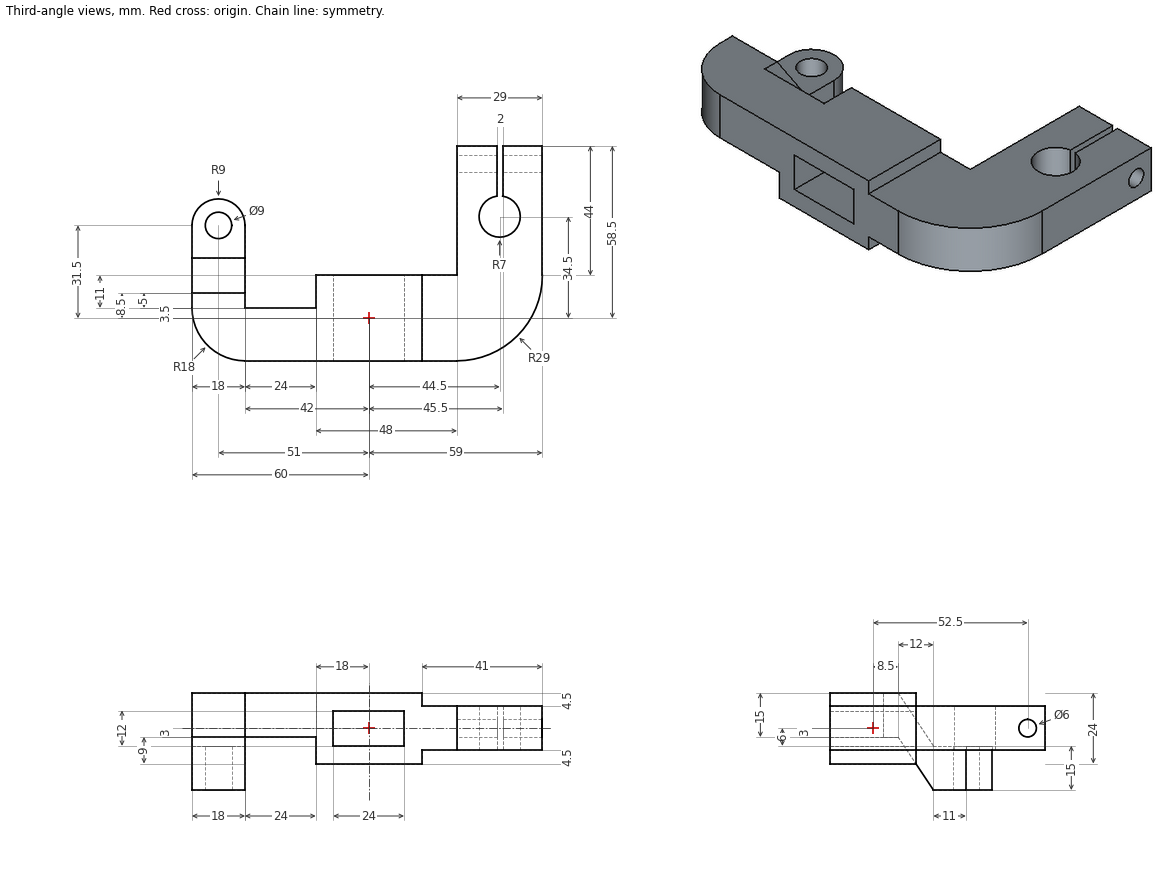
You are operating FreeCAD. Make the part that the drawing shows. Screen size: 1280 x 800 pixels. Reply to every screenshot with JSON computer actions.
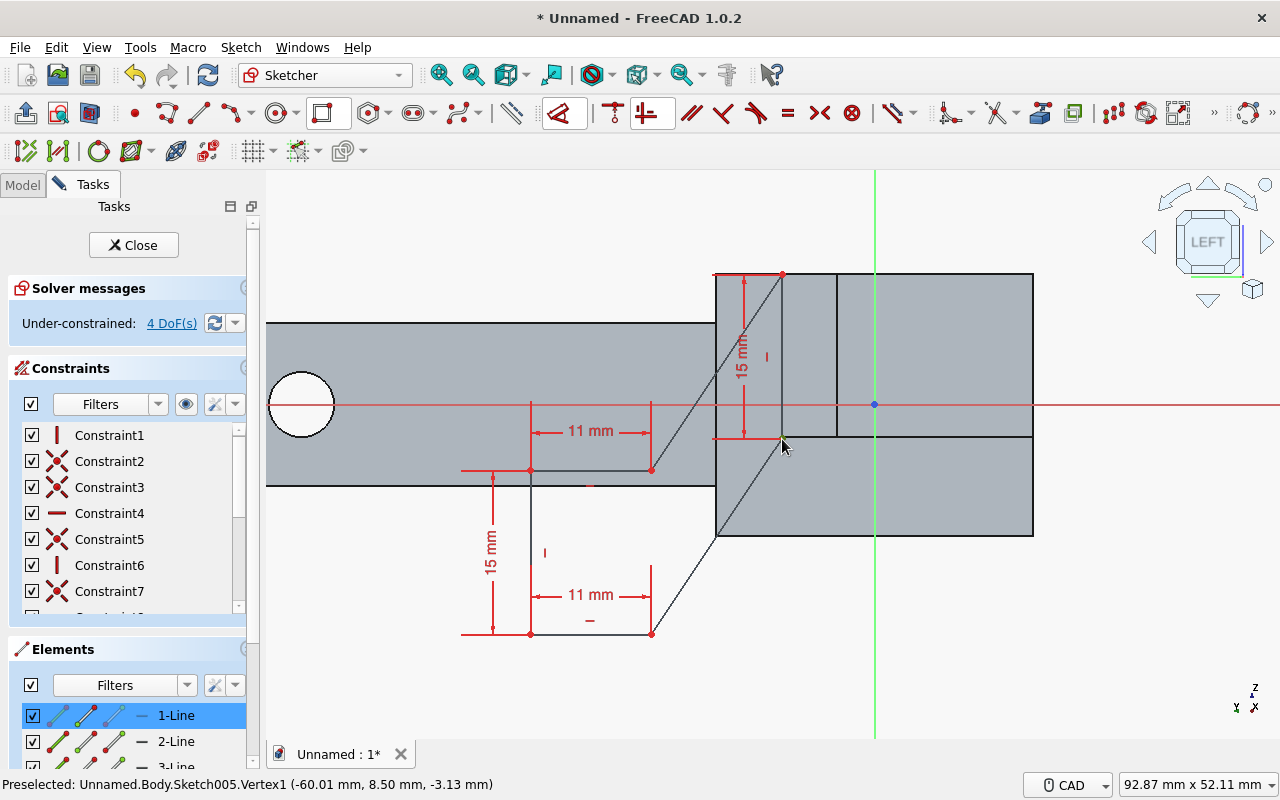
{"action": "key", "text": "i"}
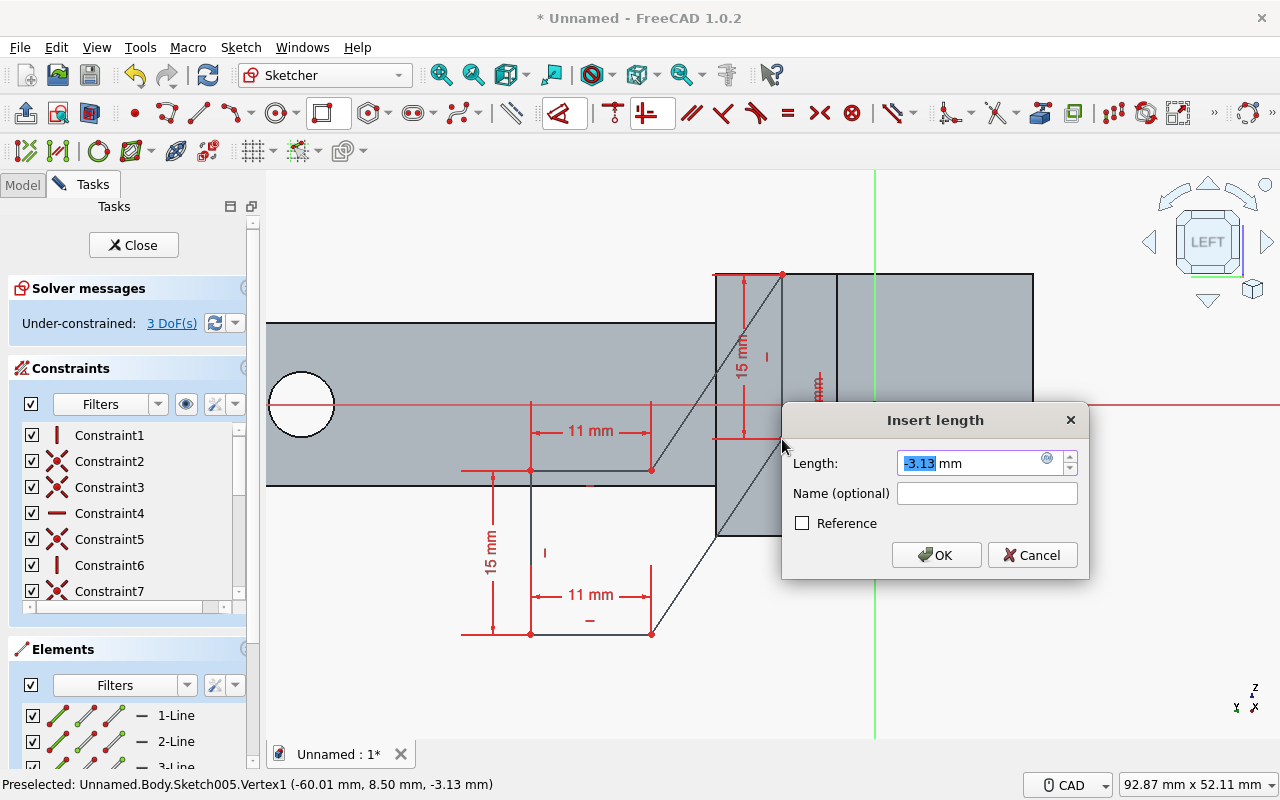
{"action": "type", "text": "-3"}
{"action": "key", "text": "Return"}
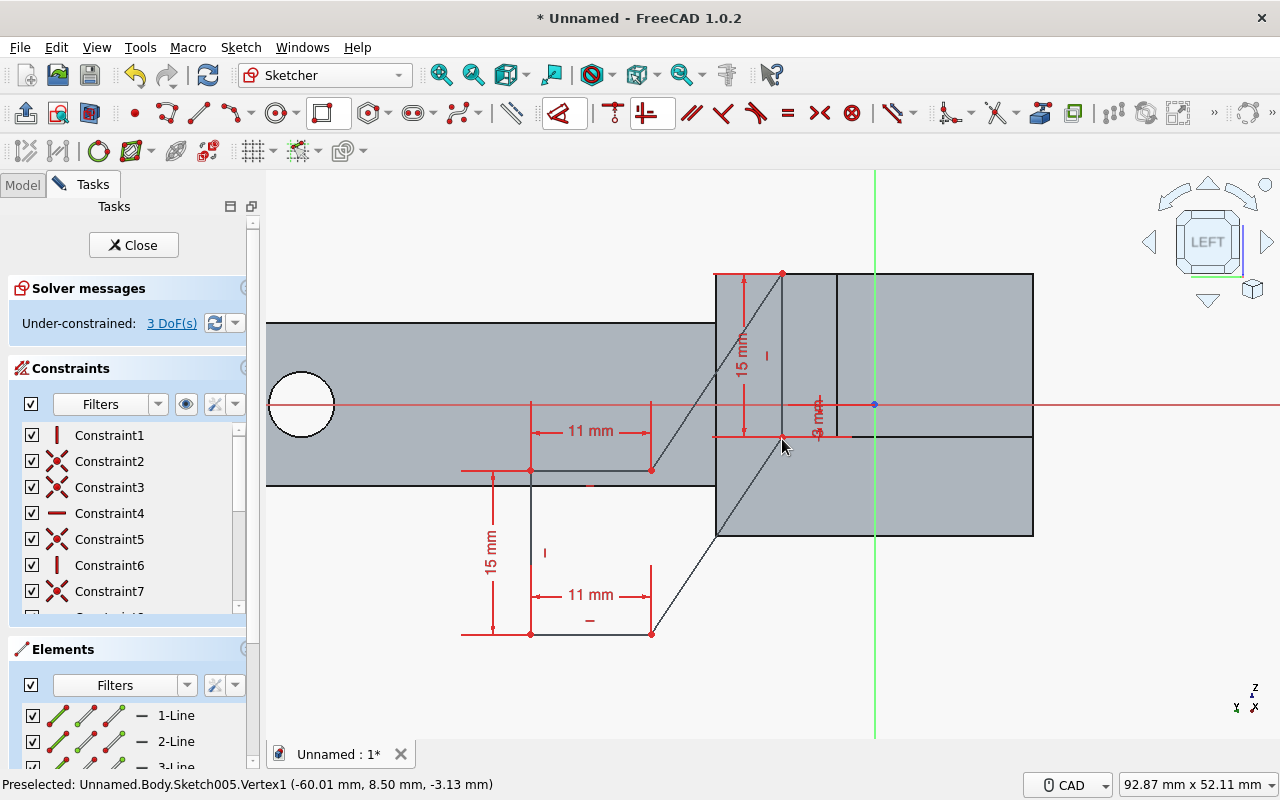
{"action": "left_click", "coordinate": [651, 471]}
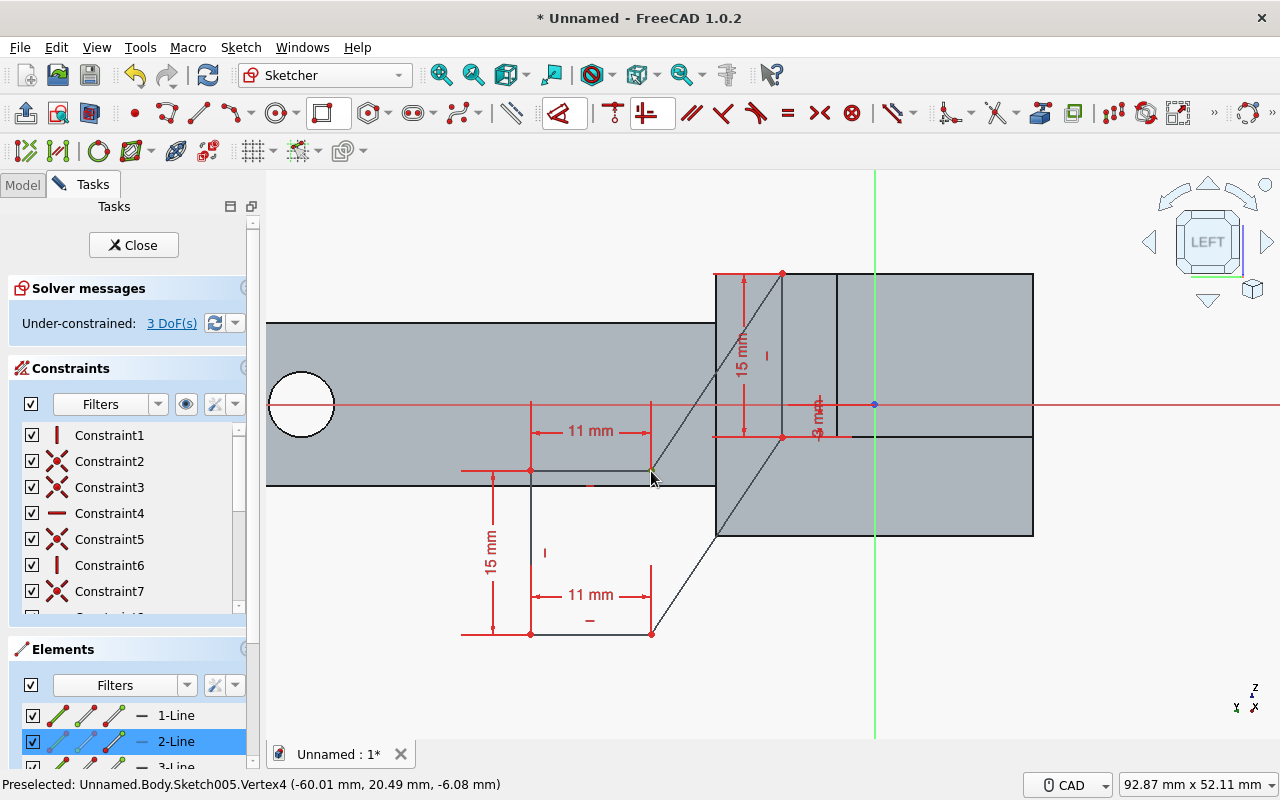
{"action": "left_click", "coordinate": [582, 114]}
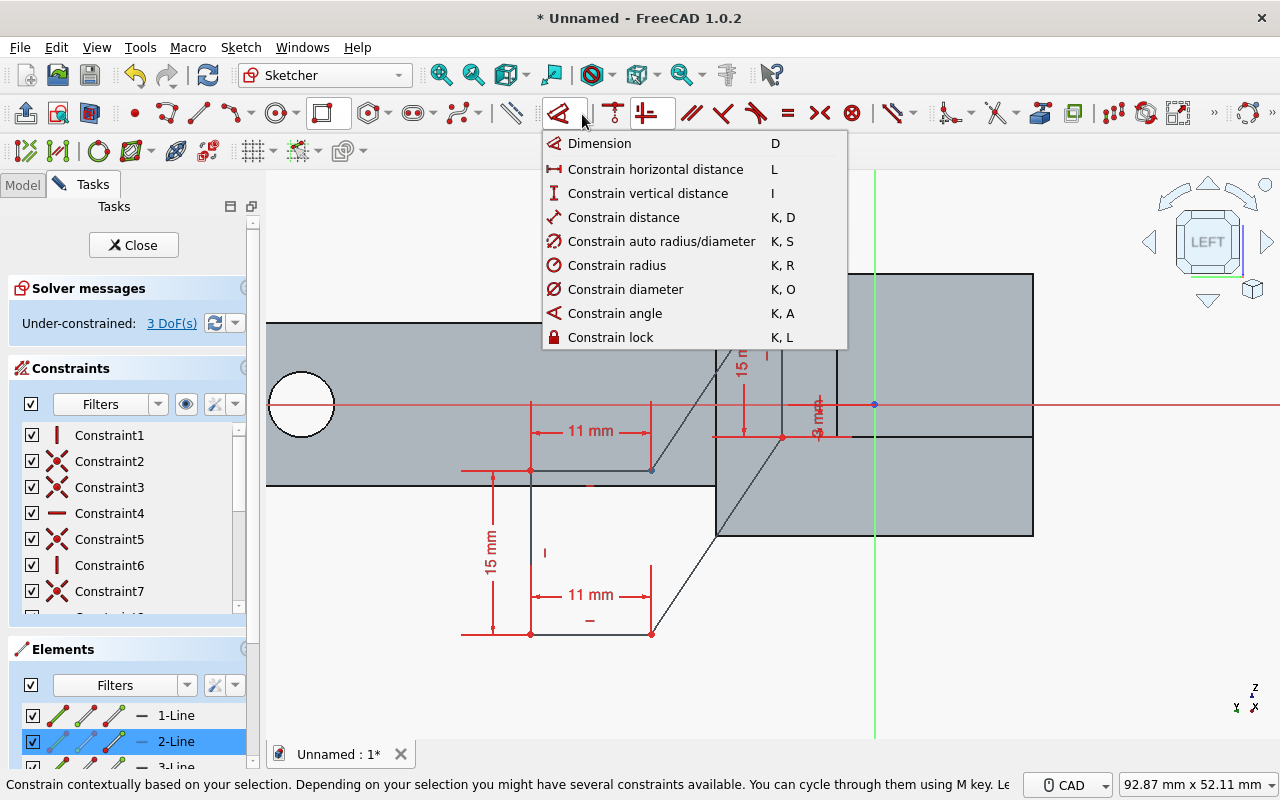
{"action": "left_click", "coordinate": [695, 193]}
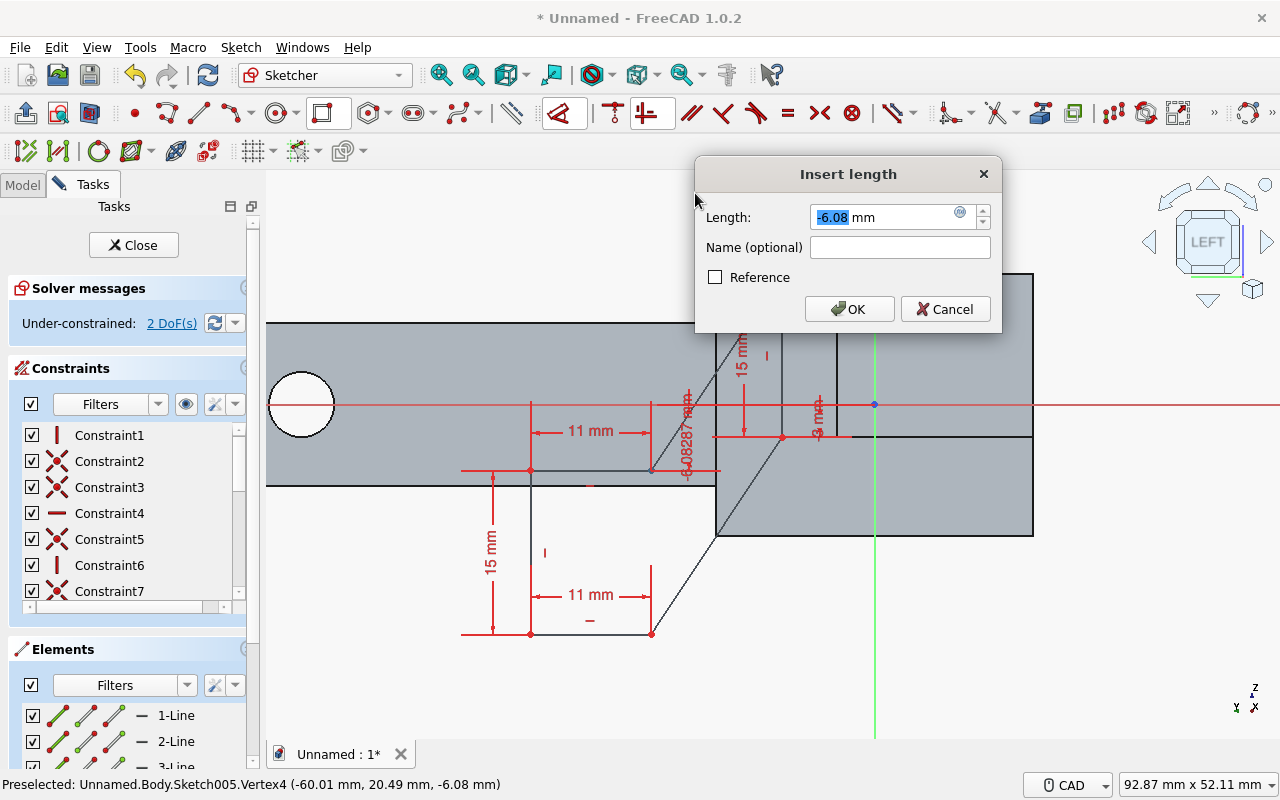
{"action": "type", "text": "-6"}
{"action": "key", "text": "Return"}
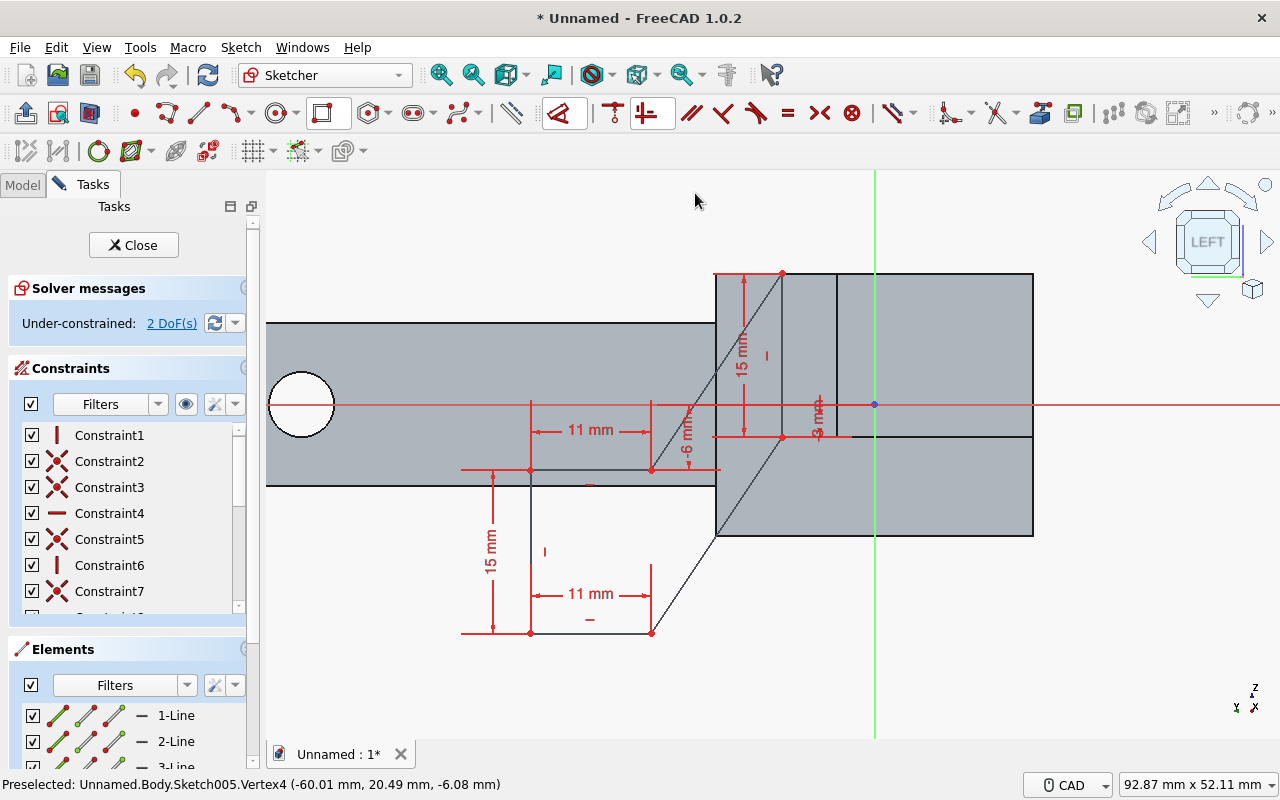
{"action": "left_click", "coordinate": [730, 352]}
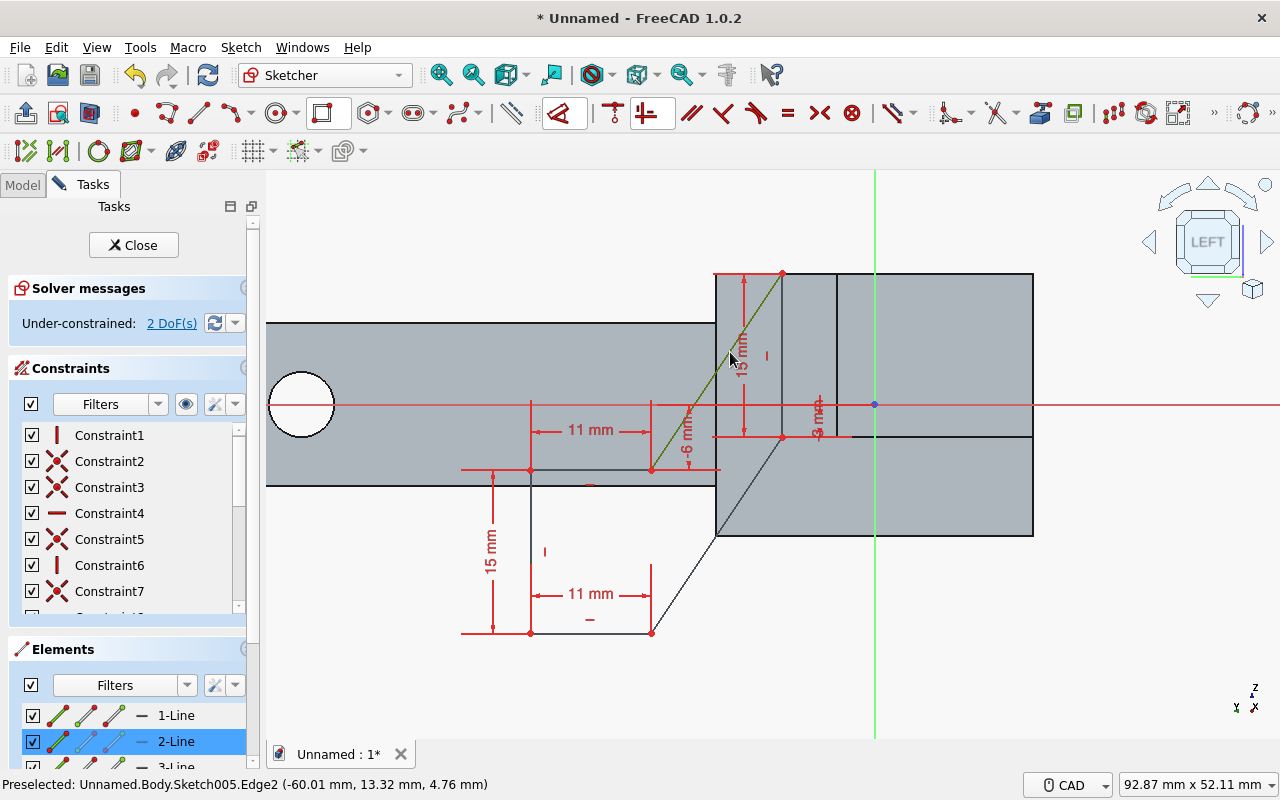
{"action": "left_click", "coordinate": [582, 114]}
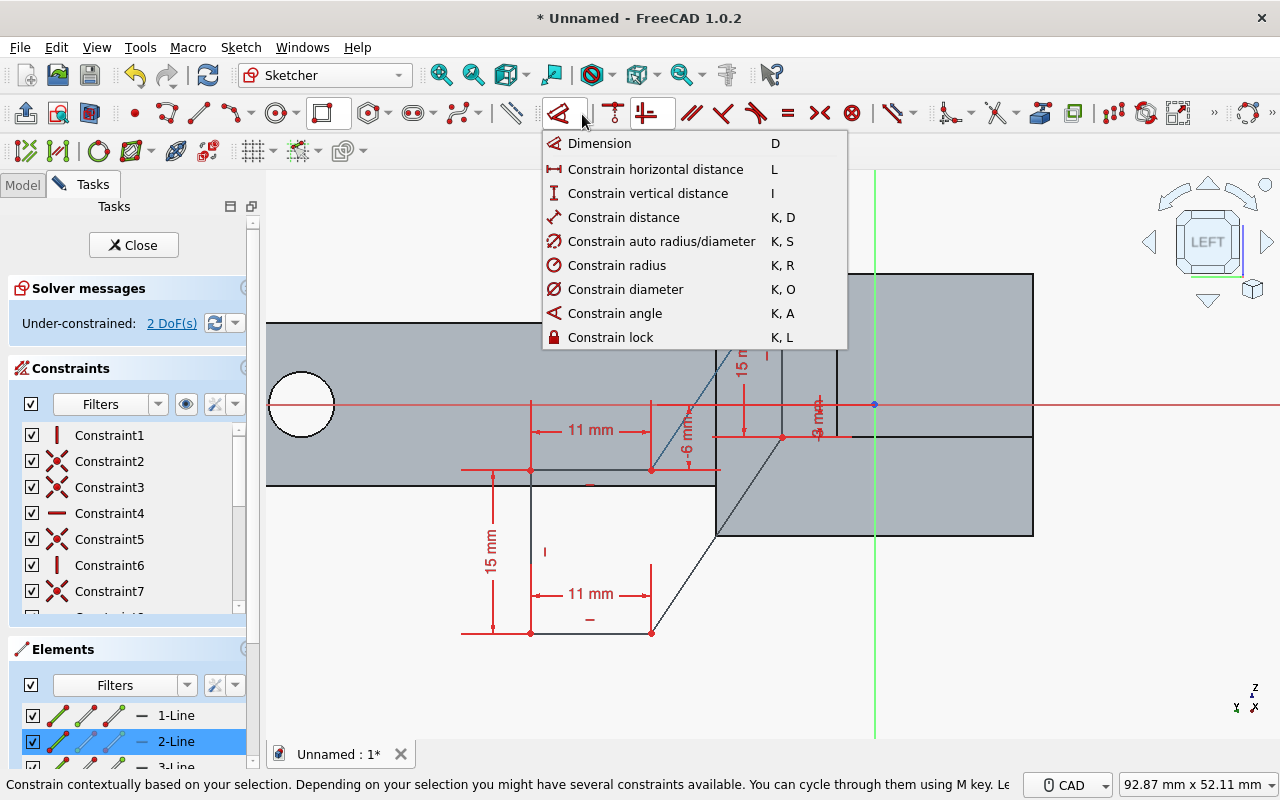
{"action": "left_click", "coordinate": [695, 169]}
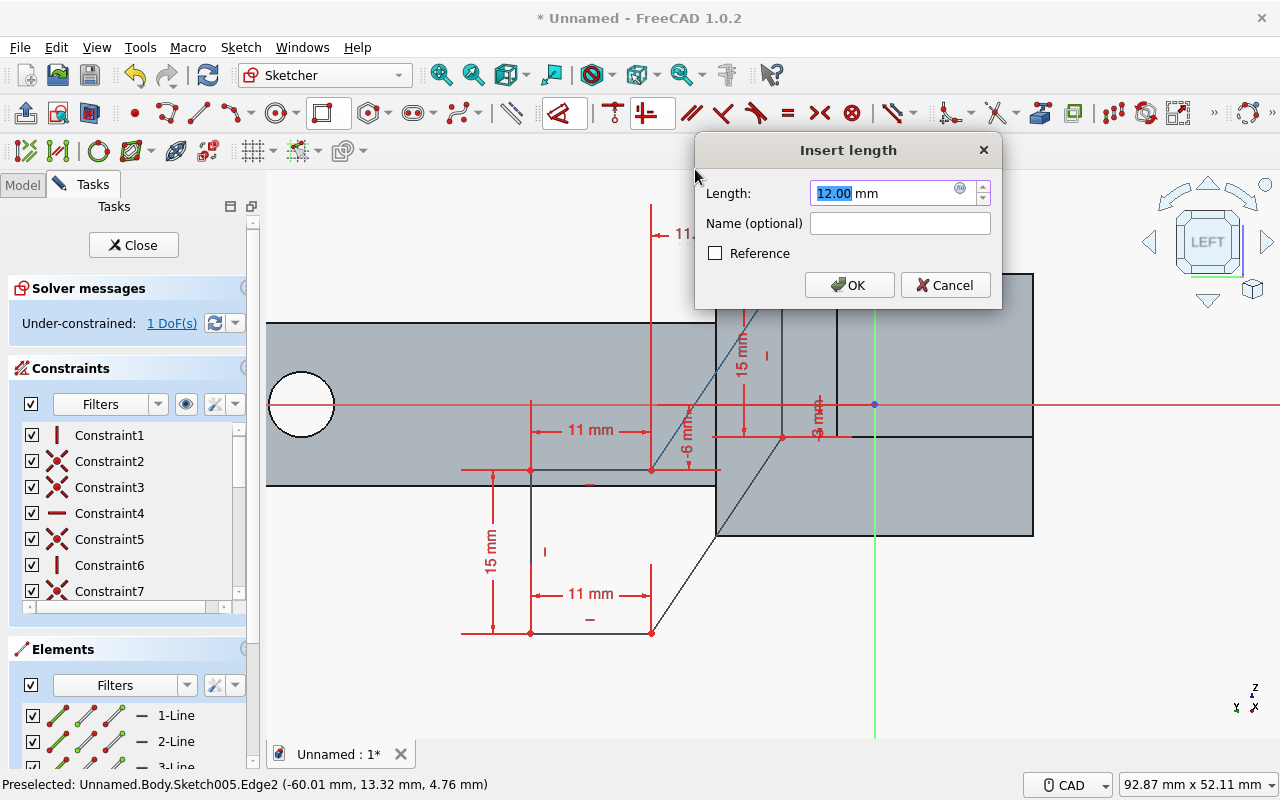
{"action": "type", "text": "12"}
{"action": "key", "text": "Return"}